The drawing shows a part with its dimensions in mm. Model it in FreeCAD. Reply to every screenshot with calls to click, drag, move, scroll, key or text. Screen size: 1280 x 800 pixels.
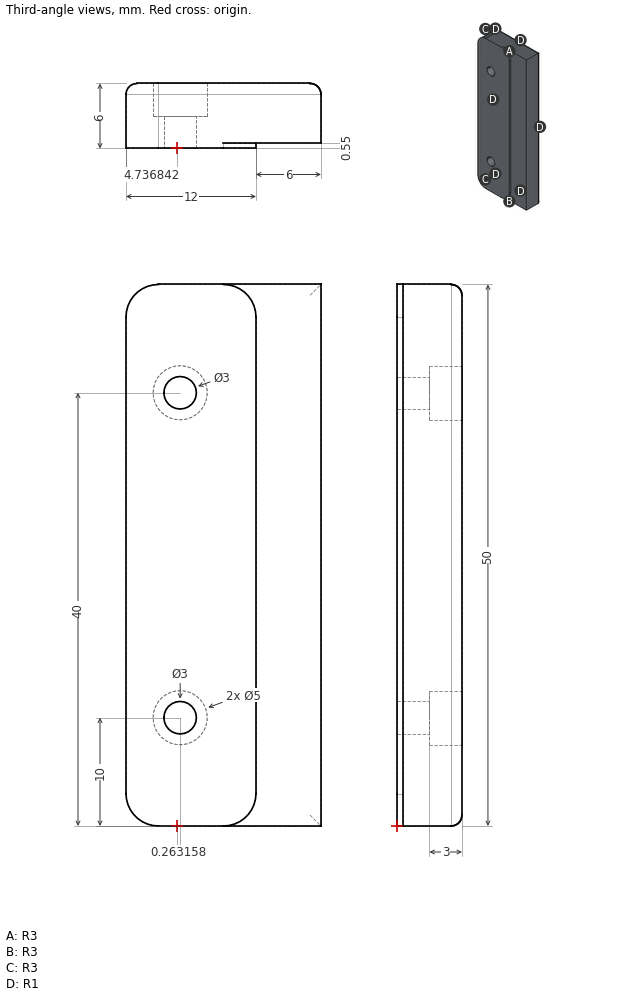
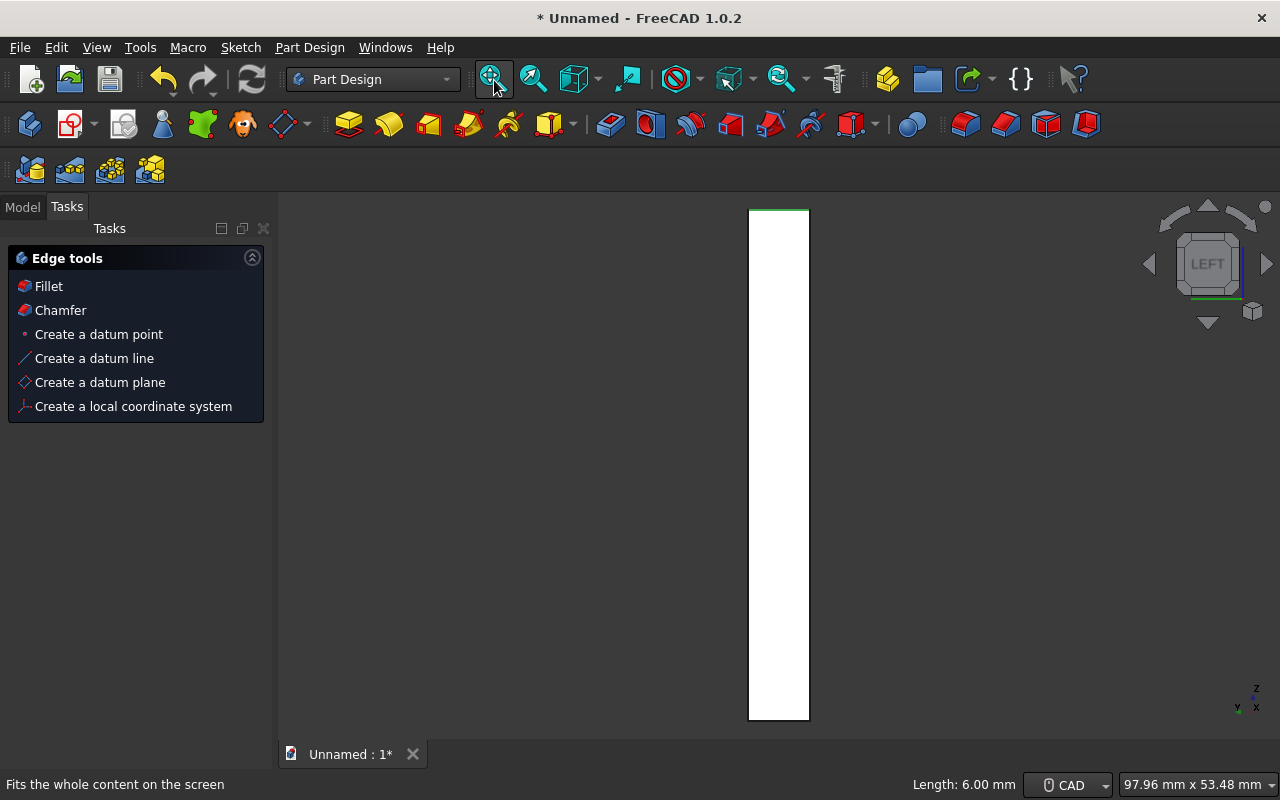
key(v)
key(3)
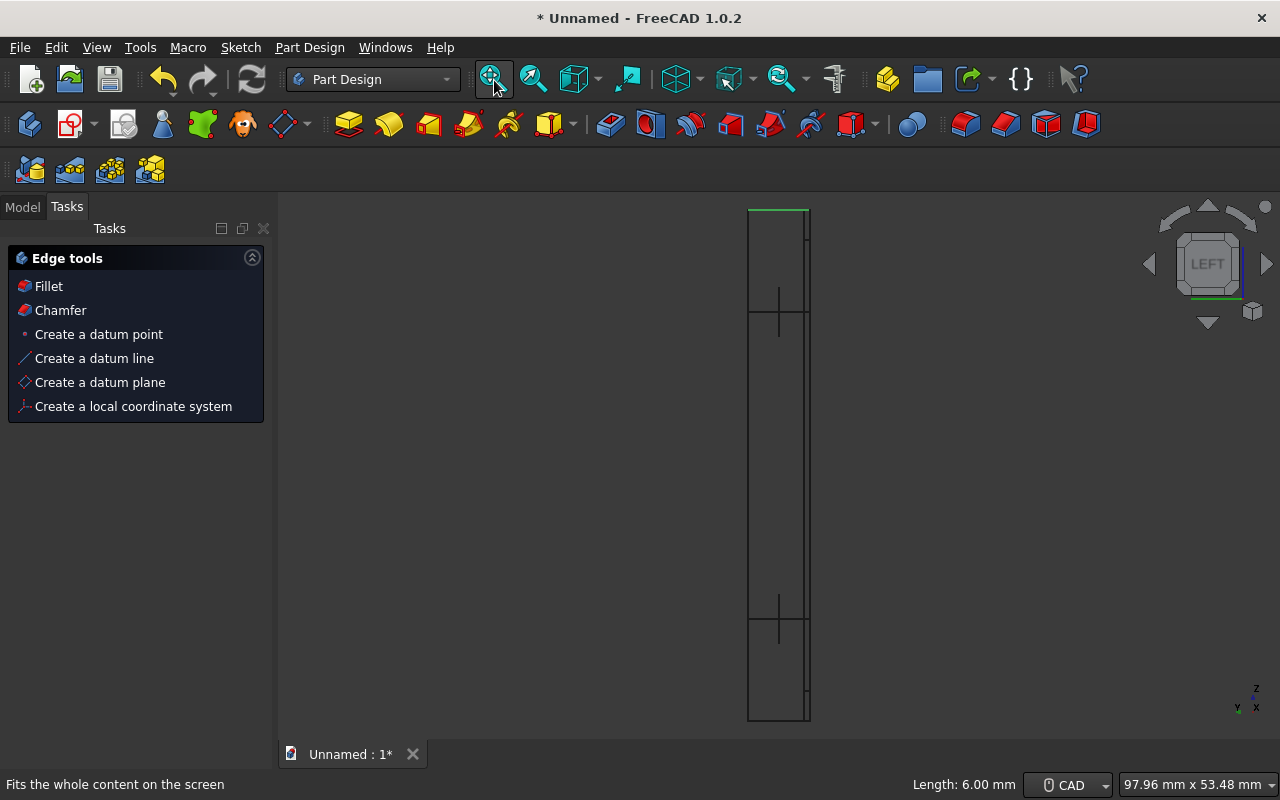
key(0)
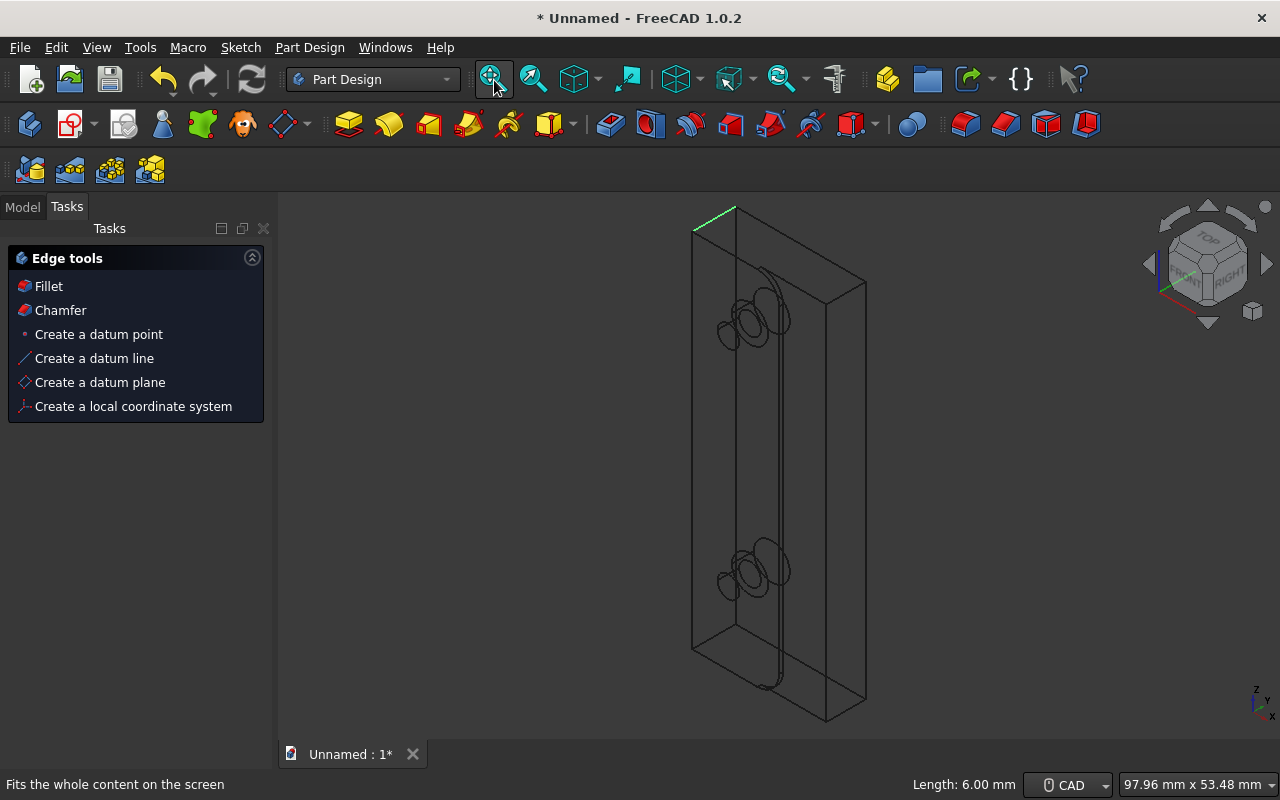
click(714, 636, ctrl)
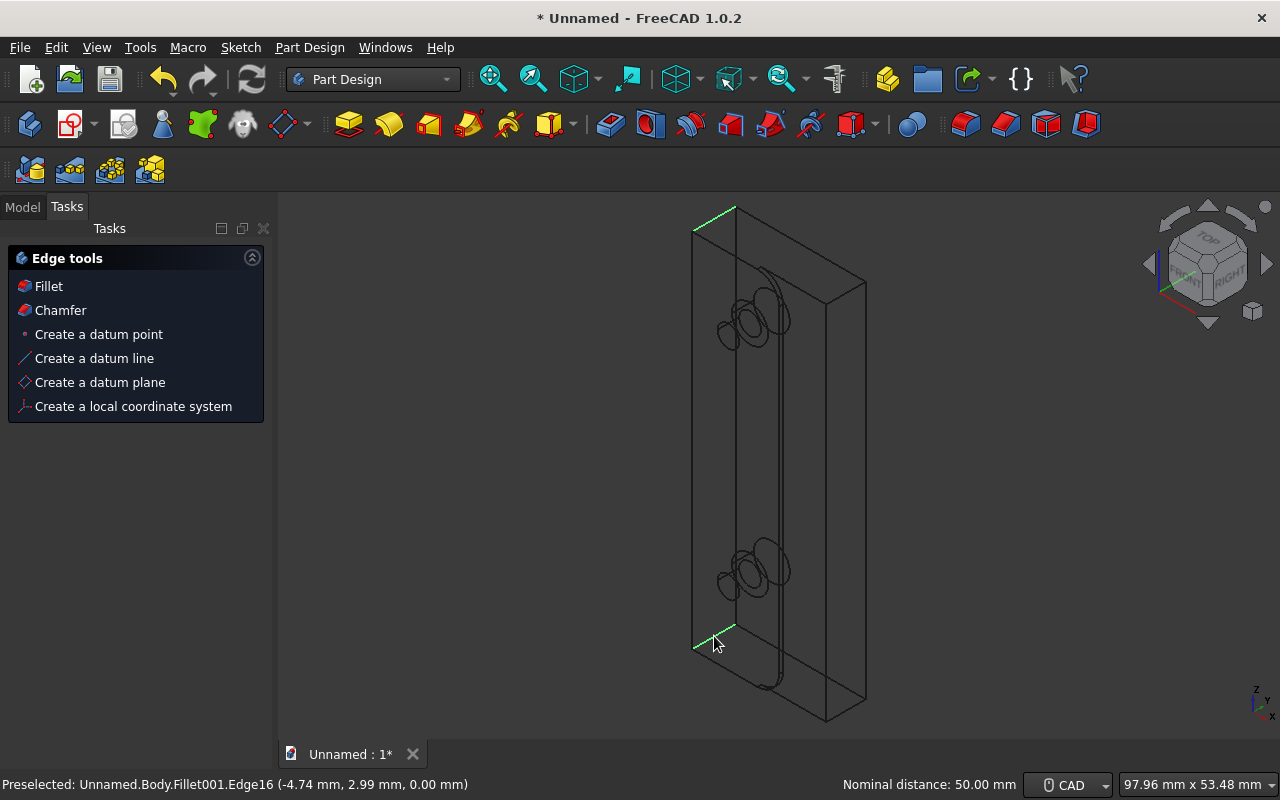
key(v)
key(1)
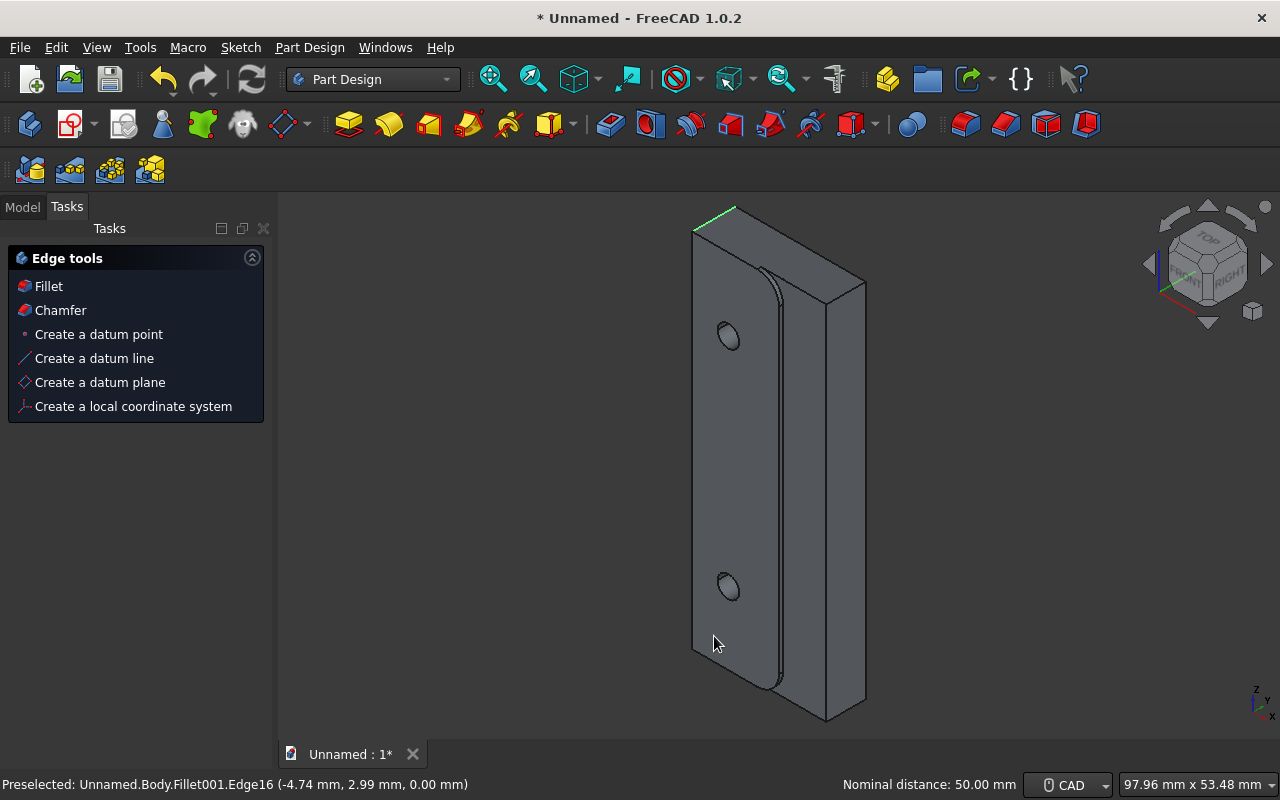
click(966, 124)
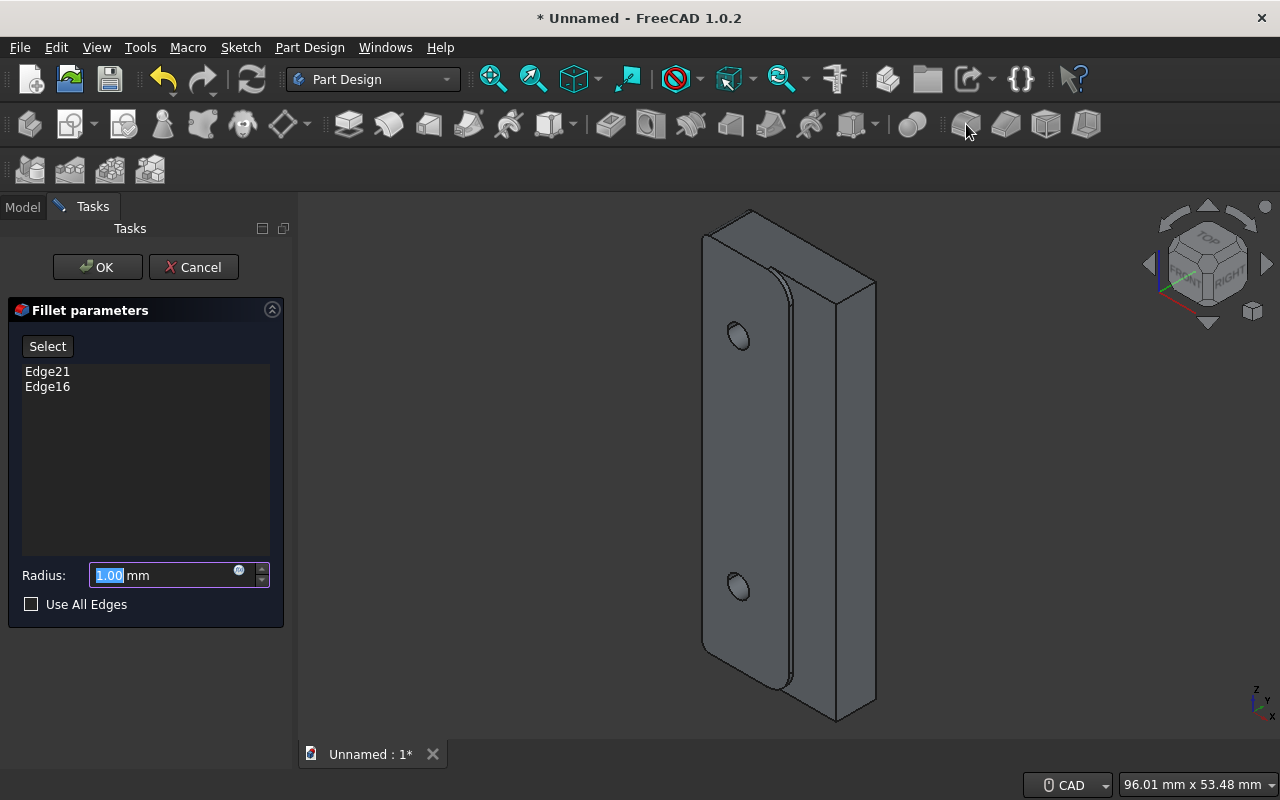
text(3)
key(Tab)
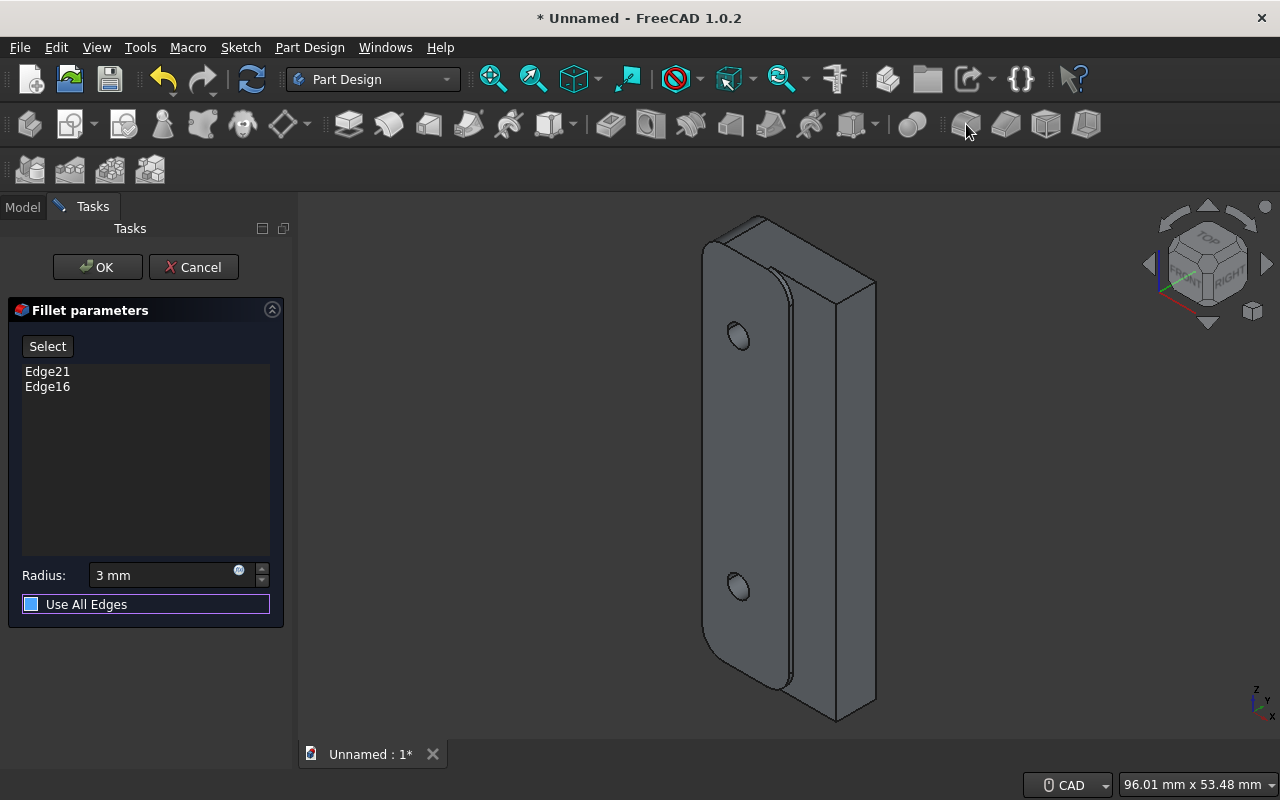
click(98, 267)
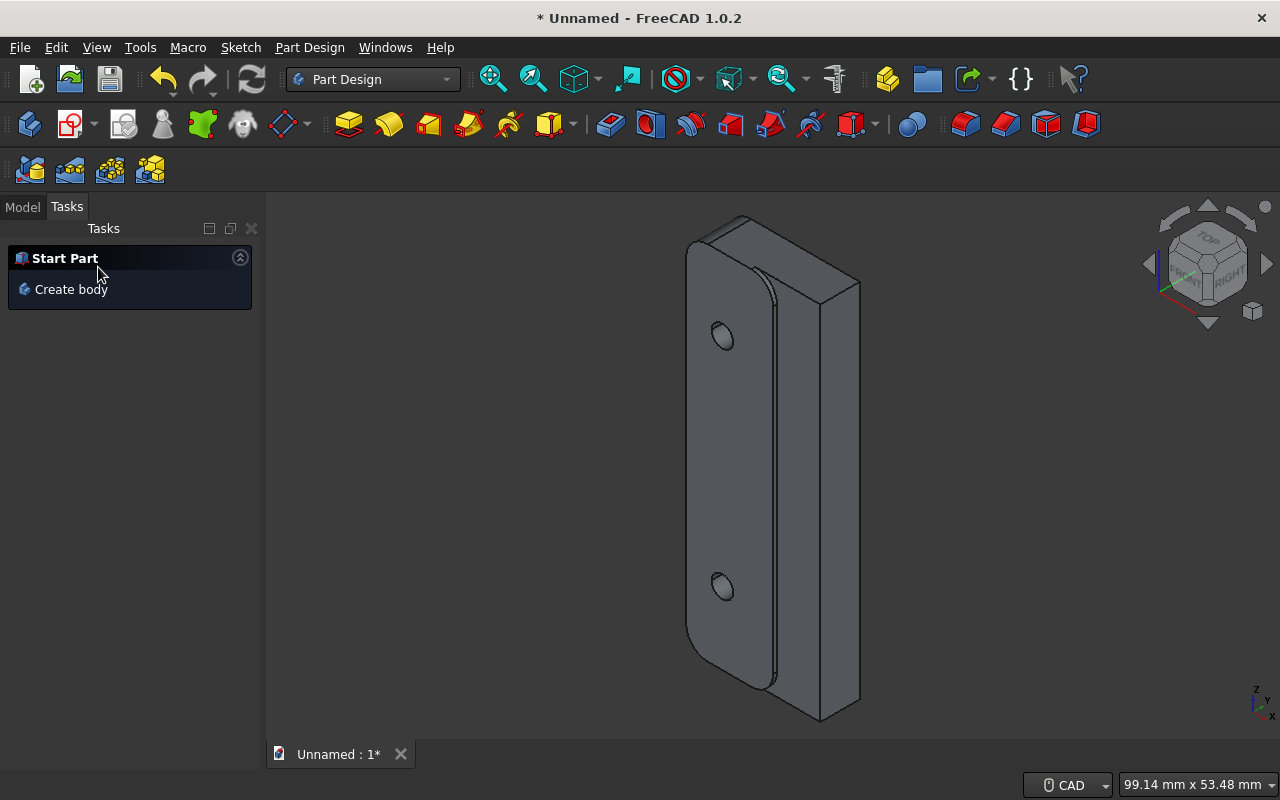
key(2)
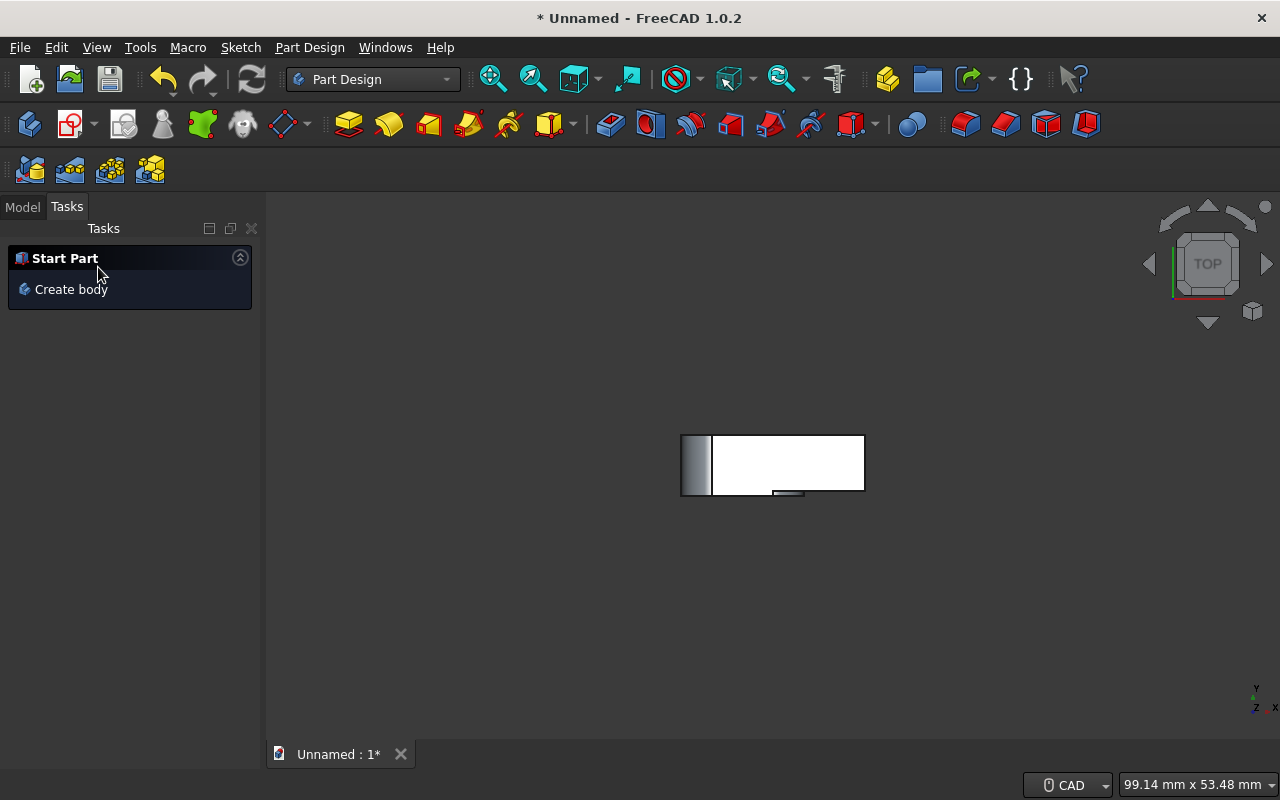
click(494, 80)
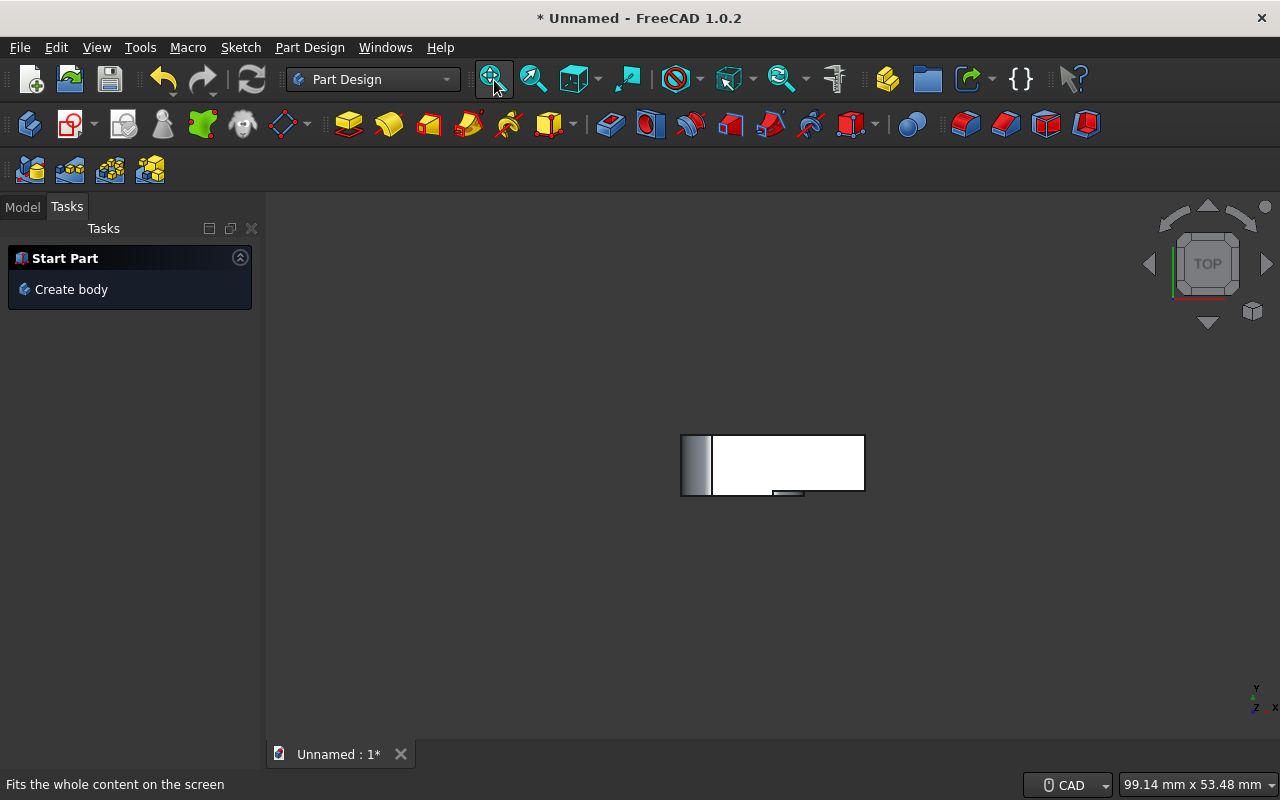
click(788, 434)